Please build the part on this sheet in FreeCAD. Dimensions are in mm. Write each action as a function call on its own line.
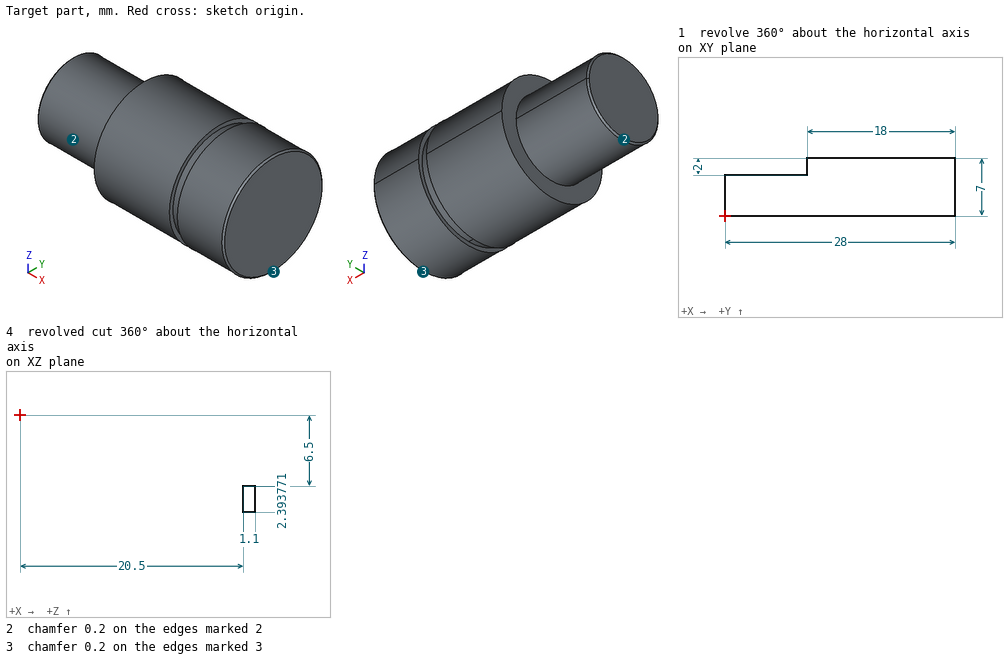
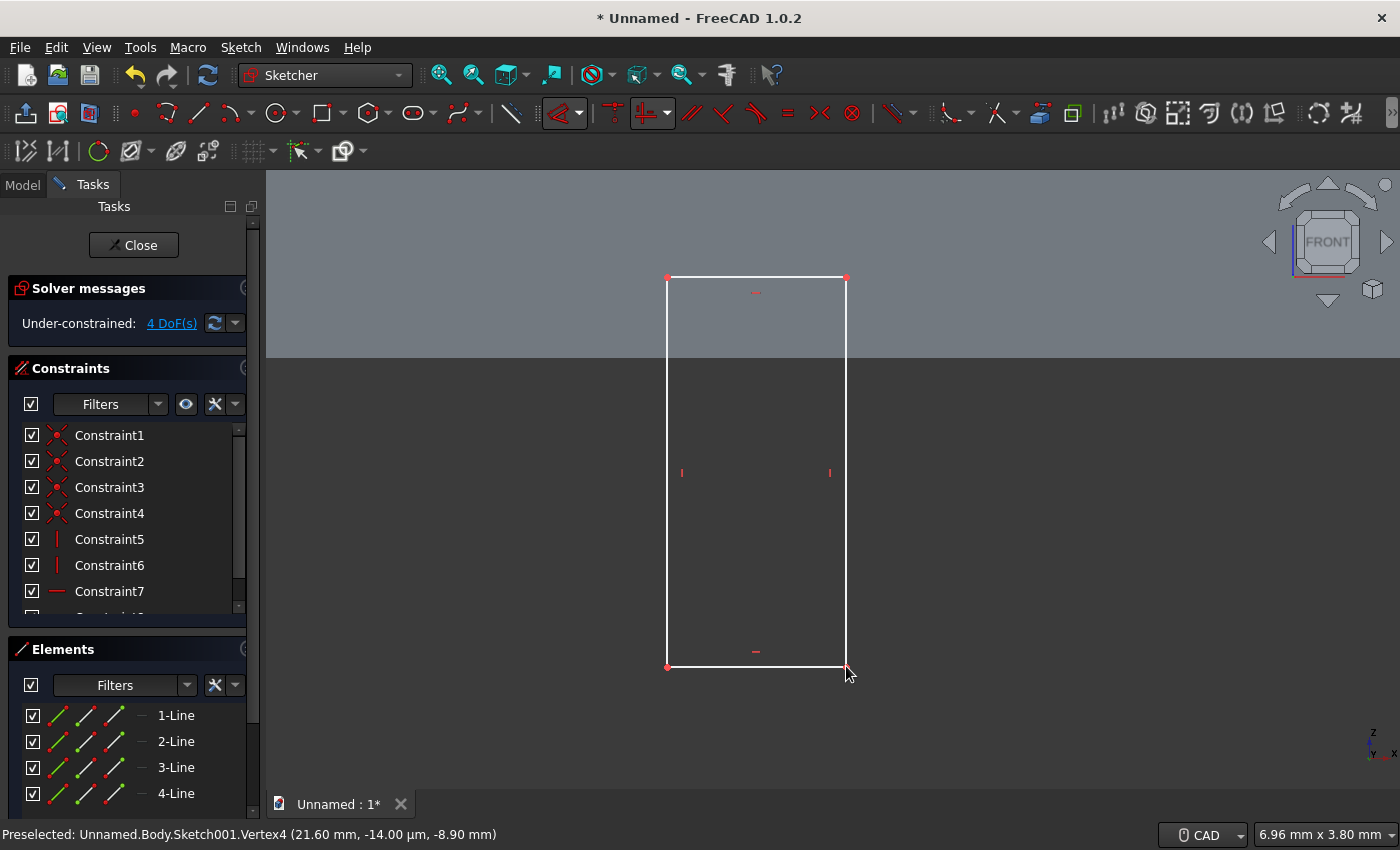
click(721, 667)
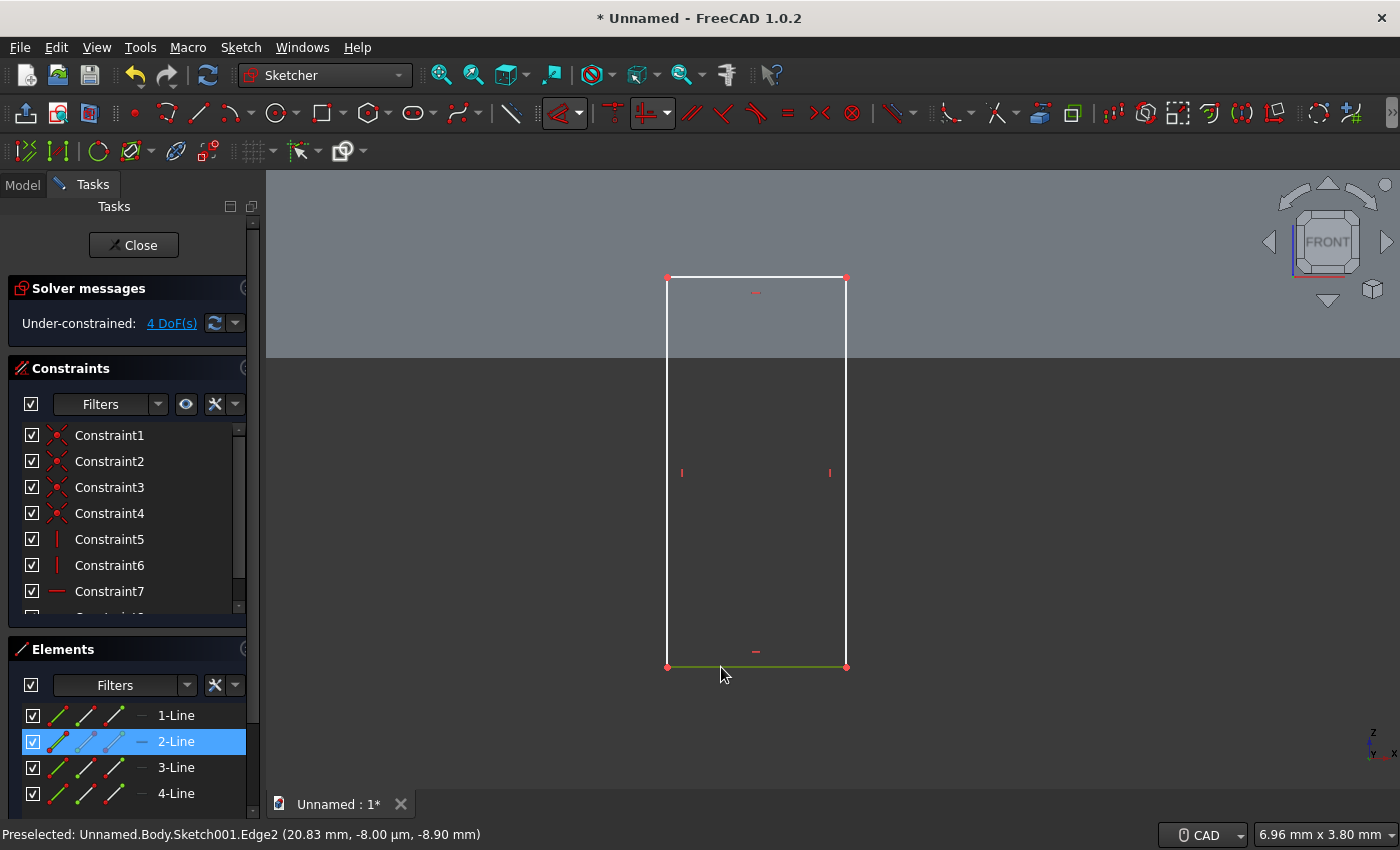
click(582, 114)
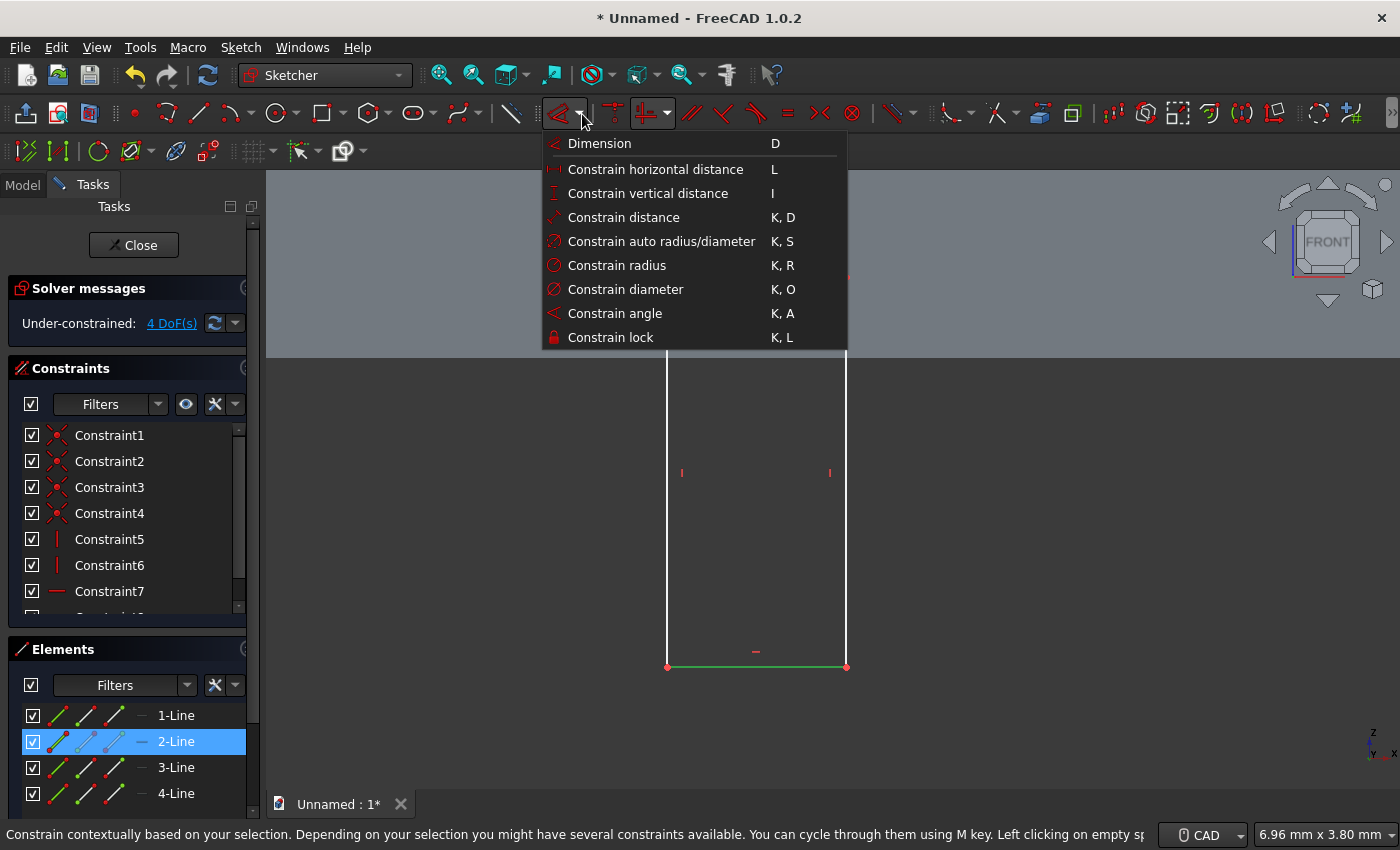
click(695, 169)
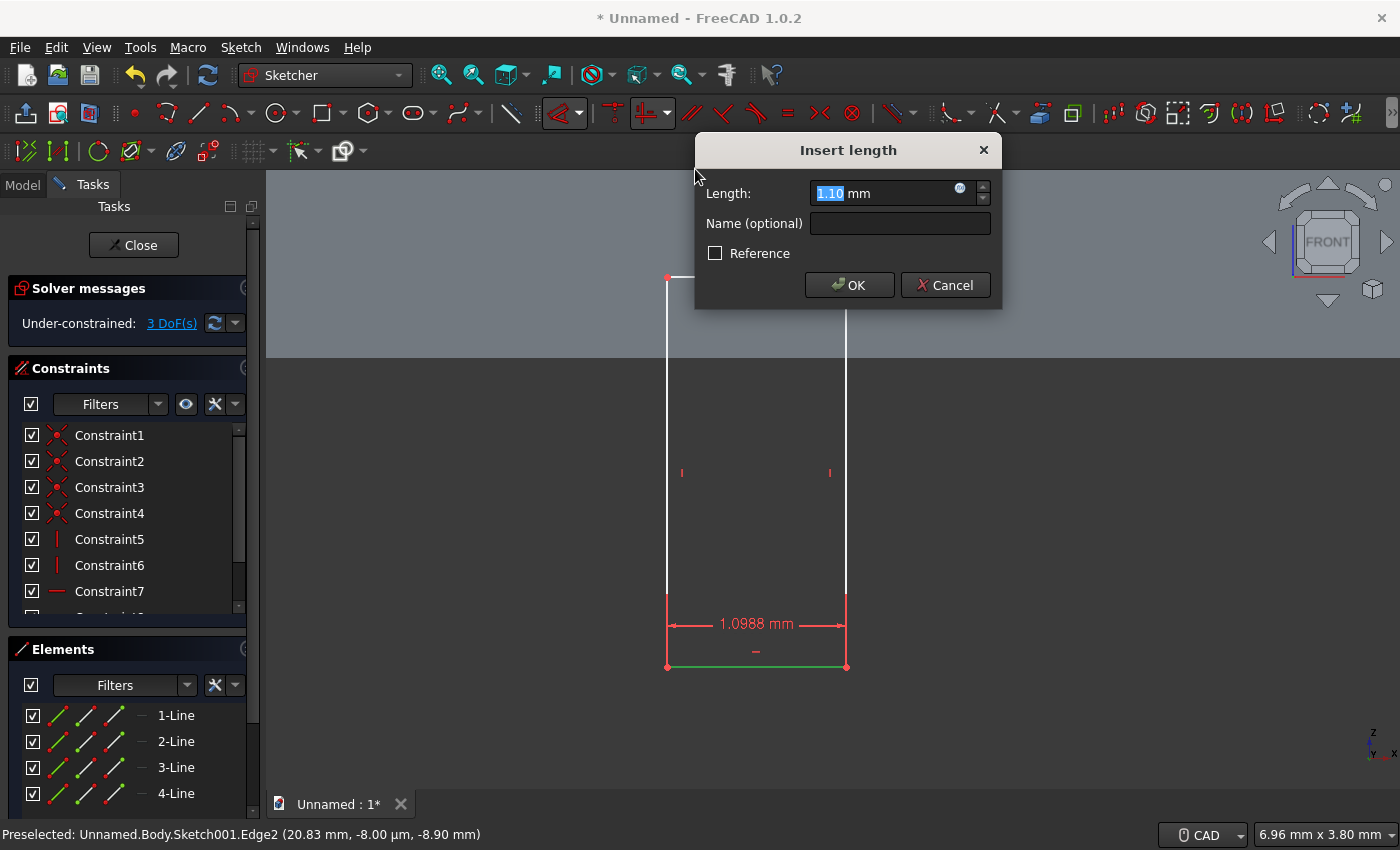
text(1.1)
key(Return)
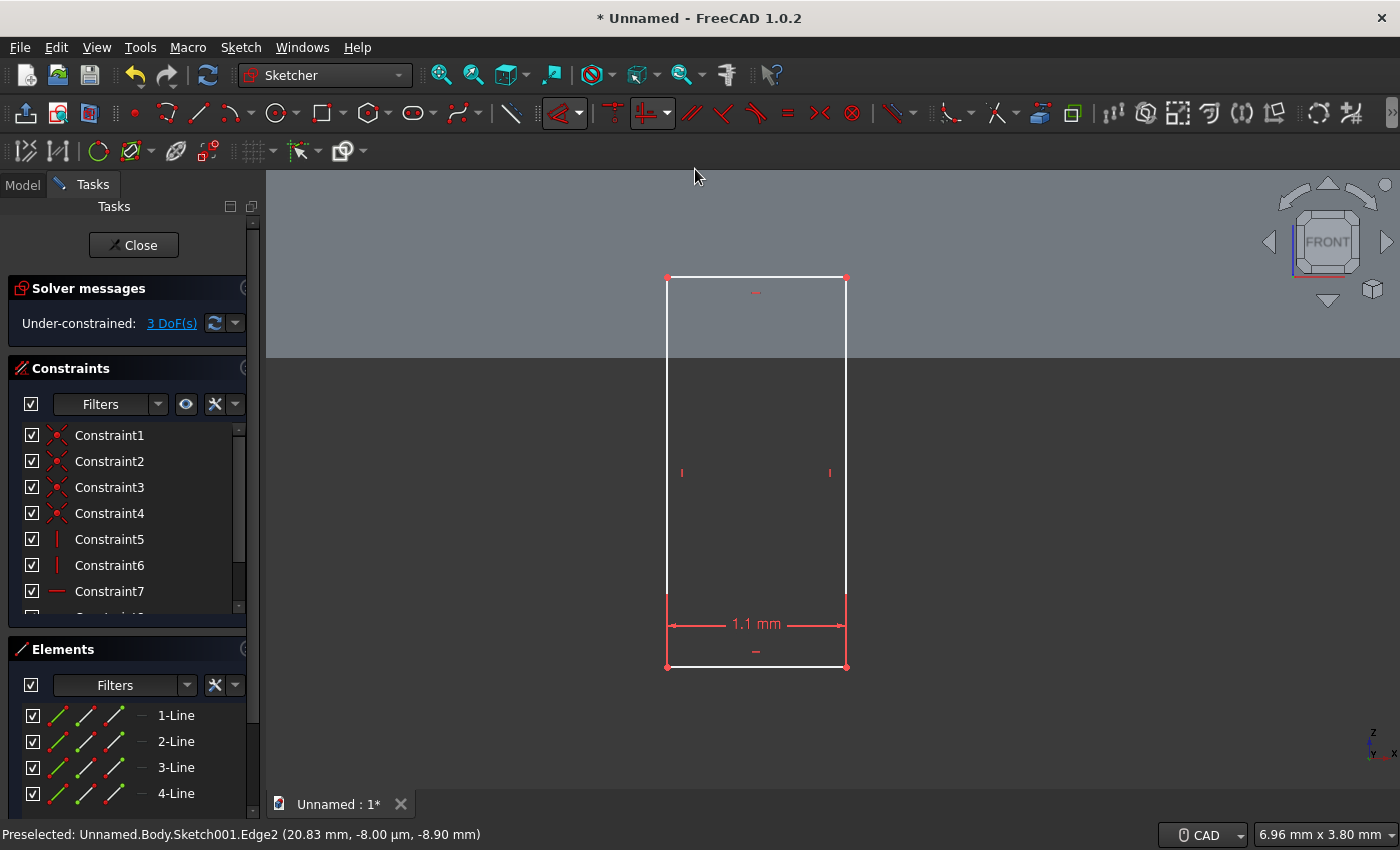
click(667, 277)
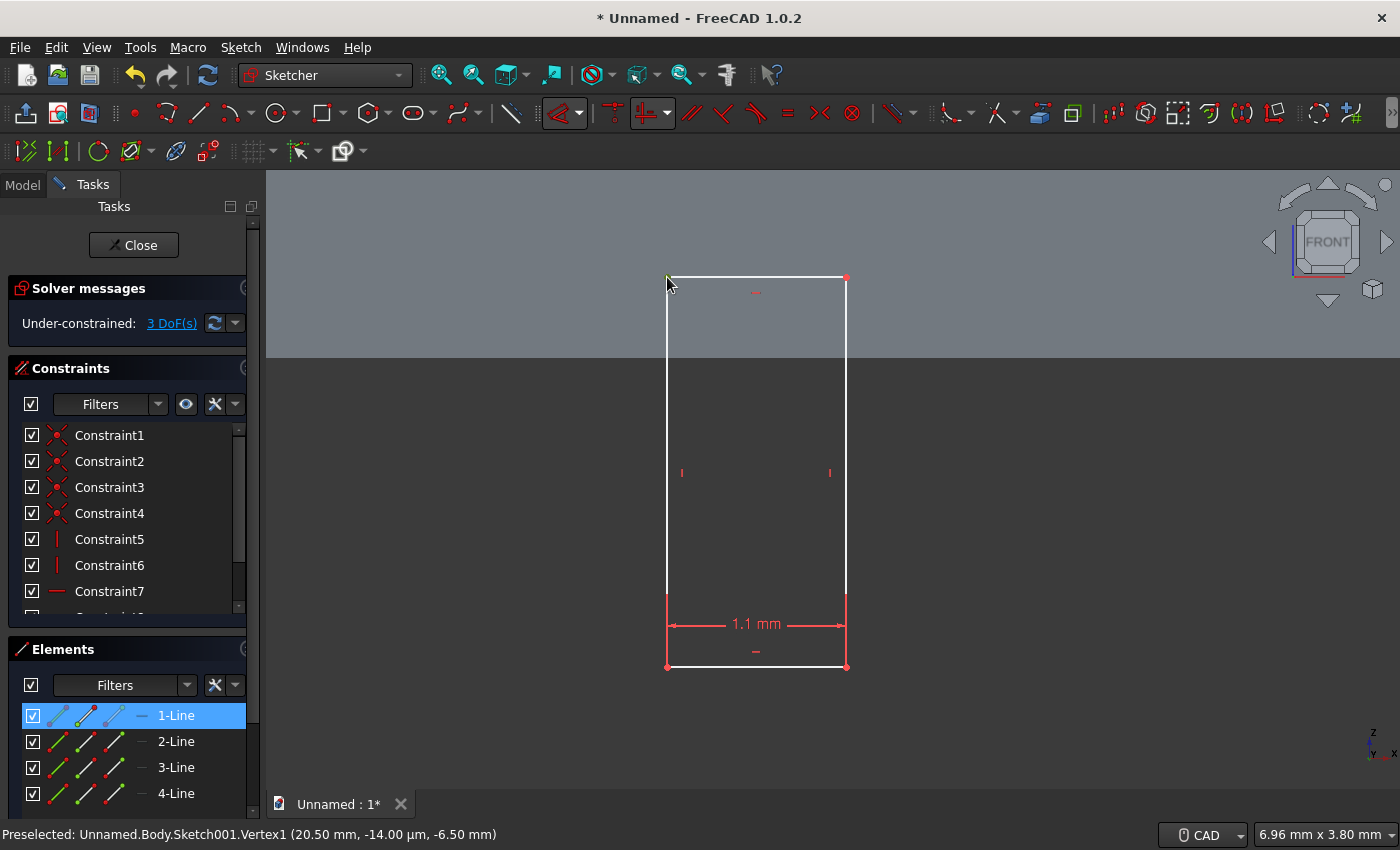
click(582, 114)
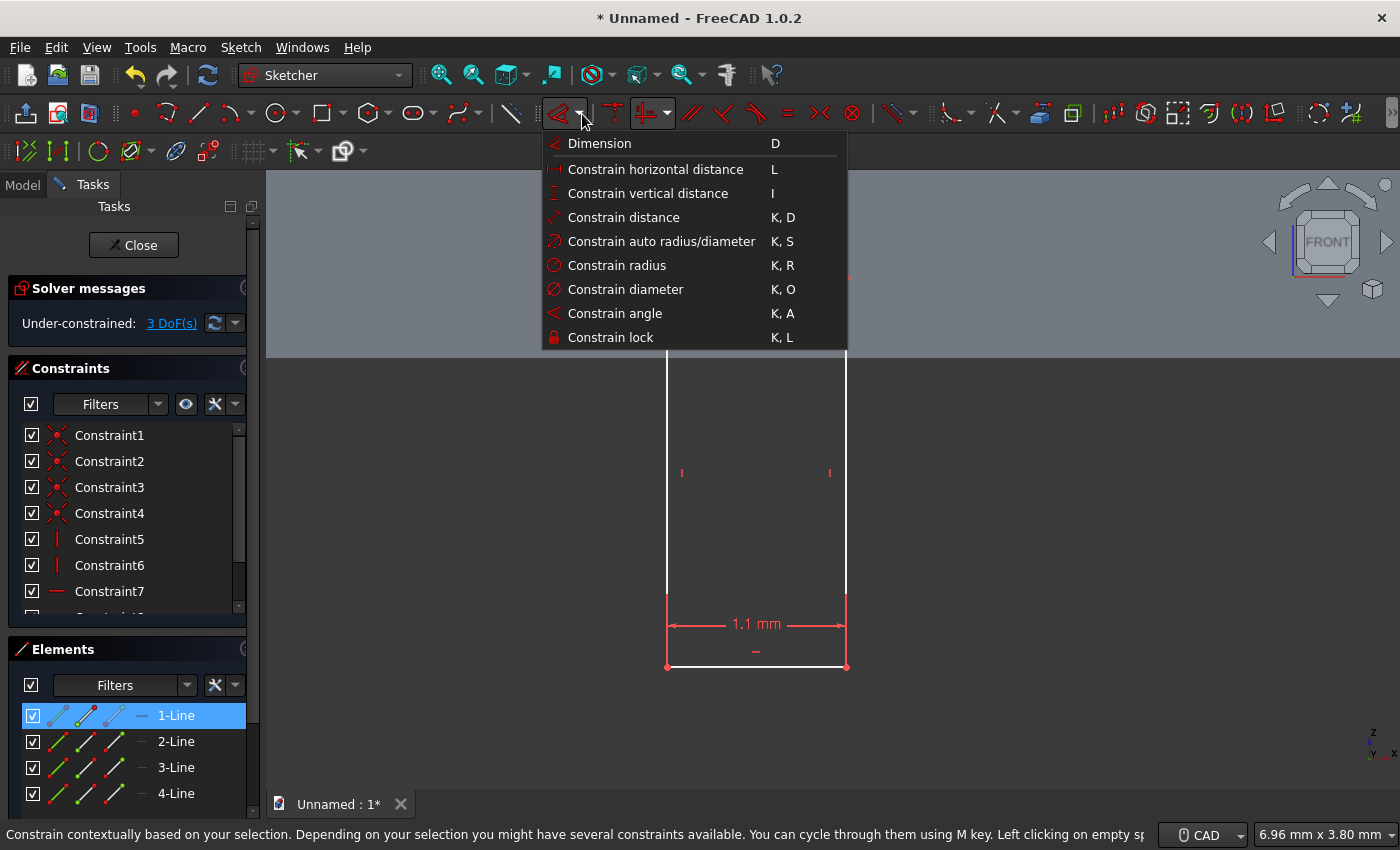
click(695, 193)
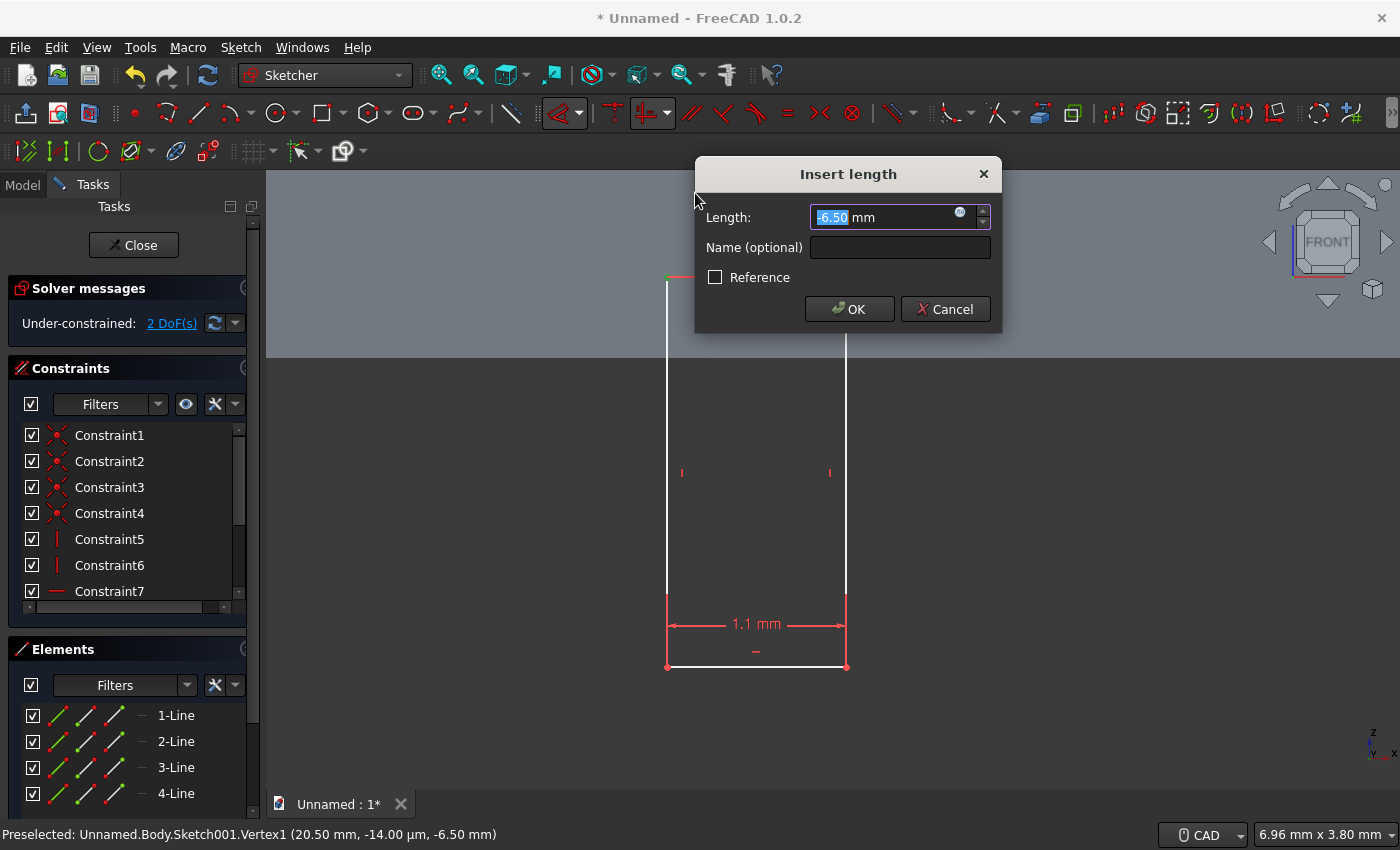
text(-6.5)
key(Return)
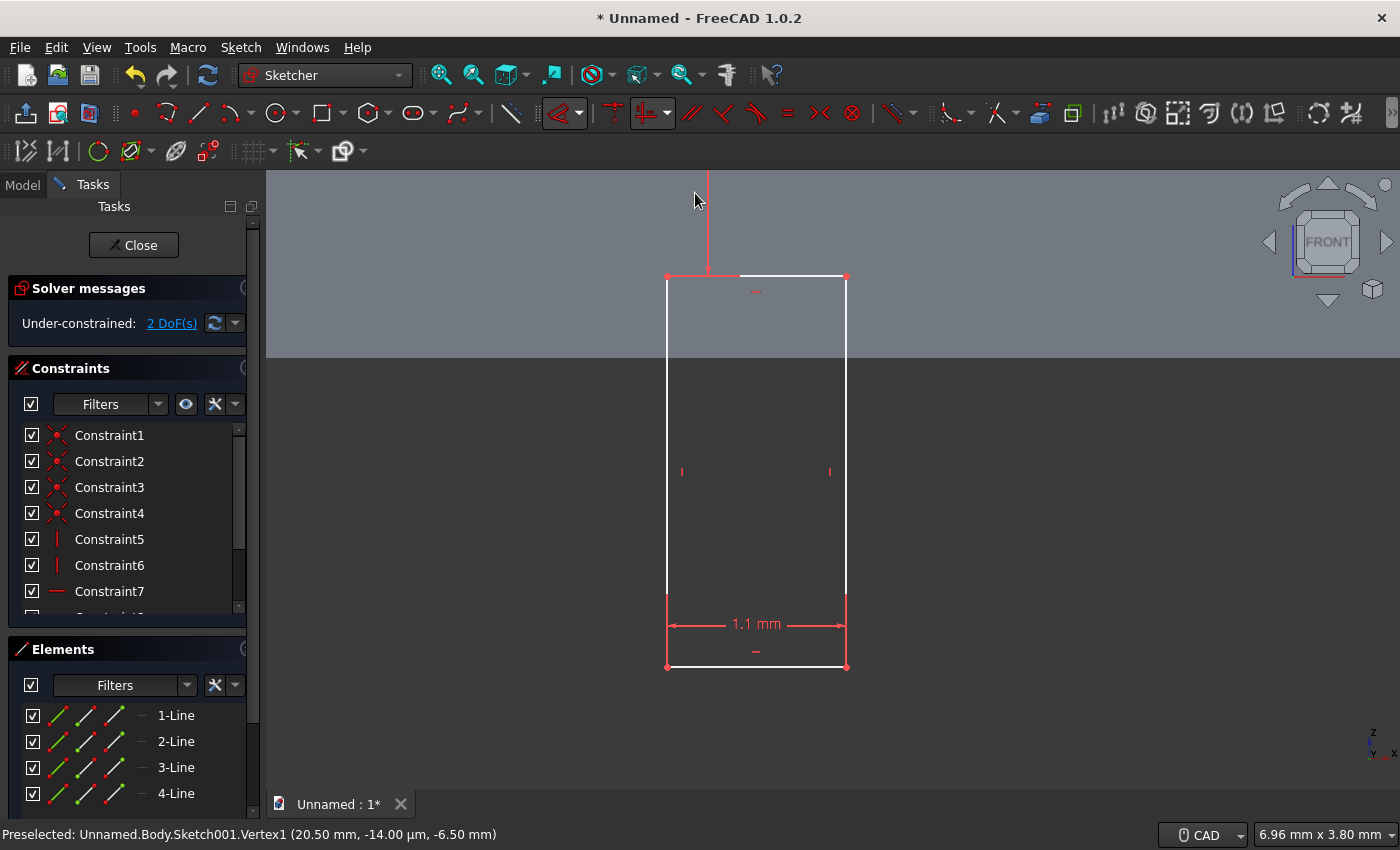
click(667, 276)